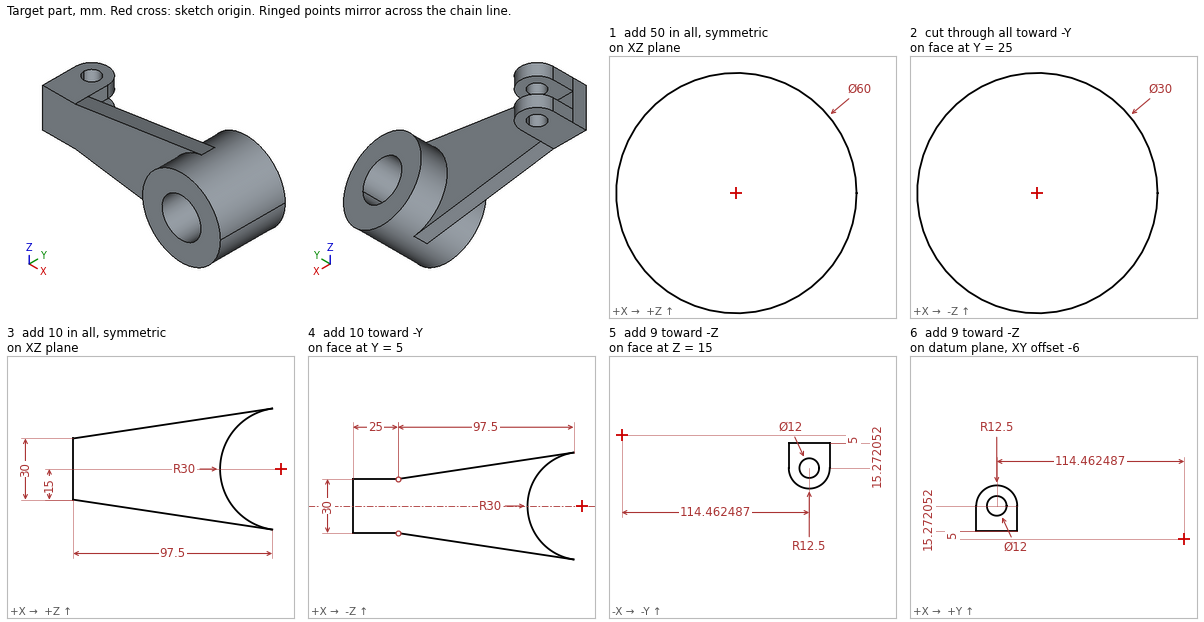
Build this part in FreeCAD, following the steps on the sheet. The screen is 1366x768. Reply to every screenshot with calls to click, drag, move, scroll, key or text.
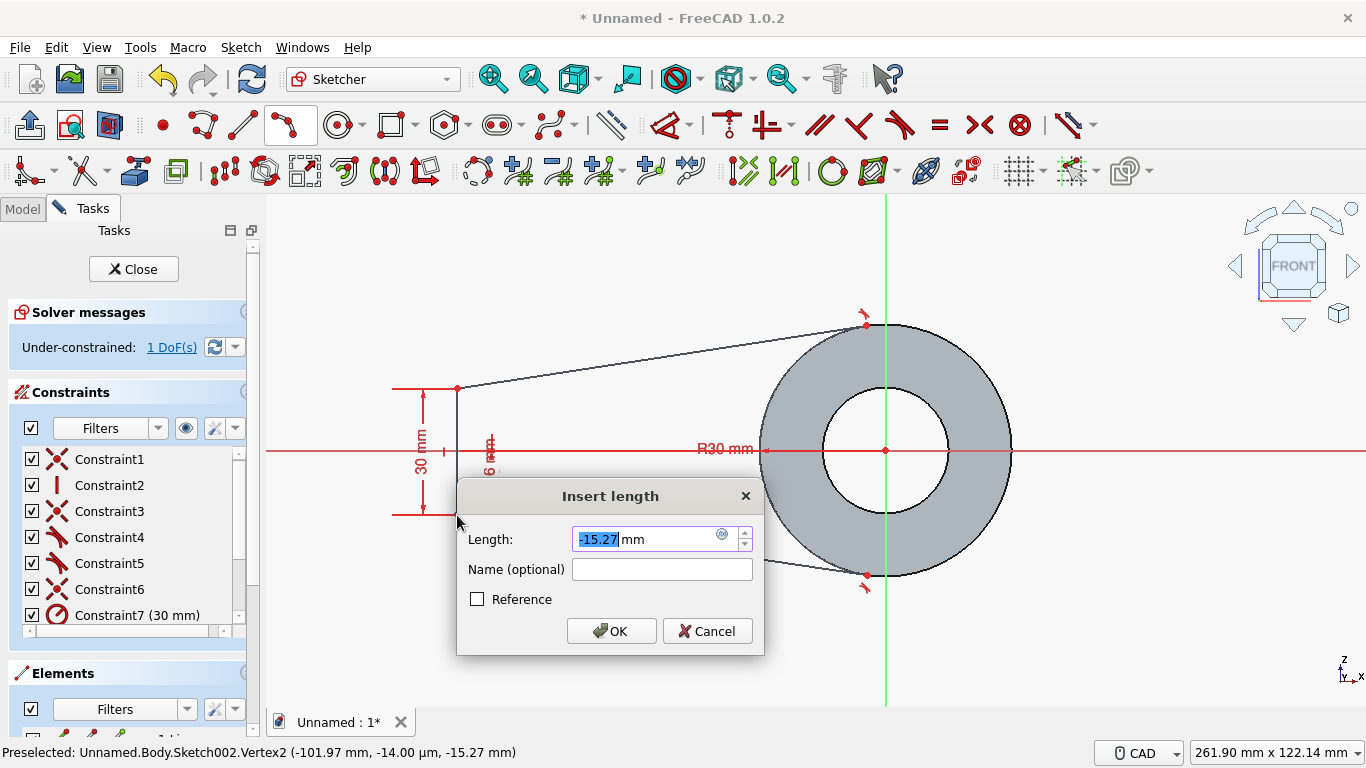
text(-15)
key(Return)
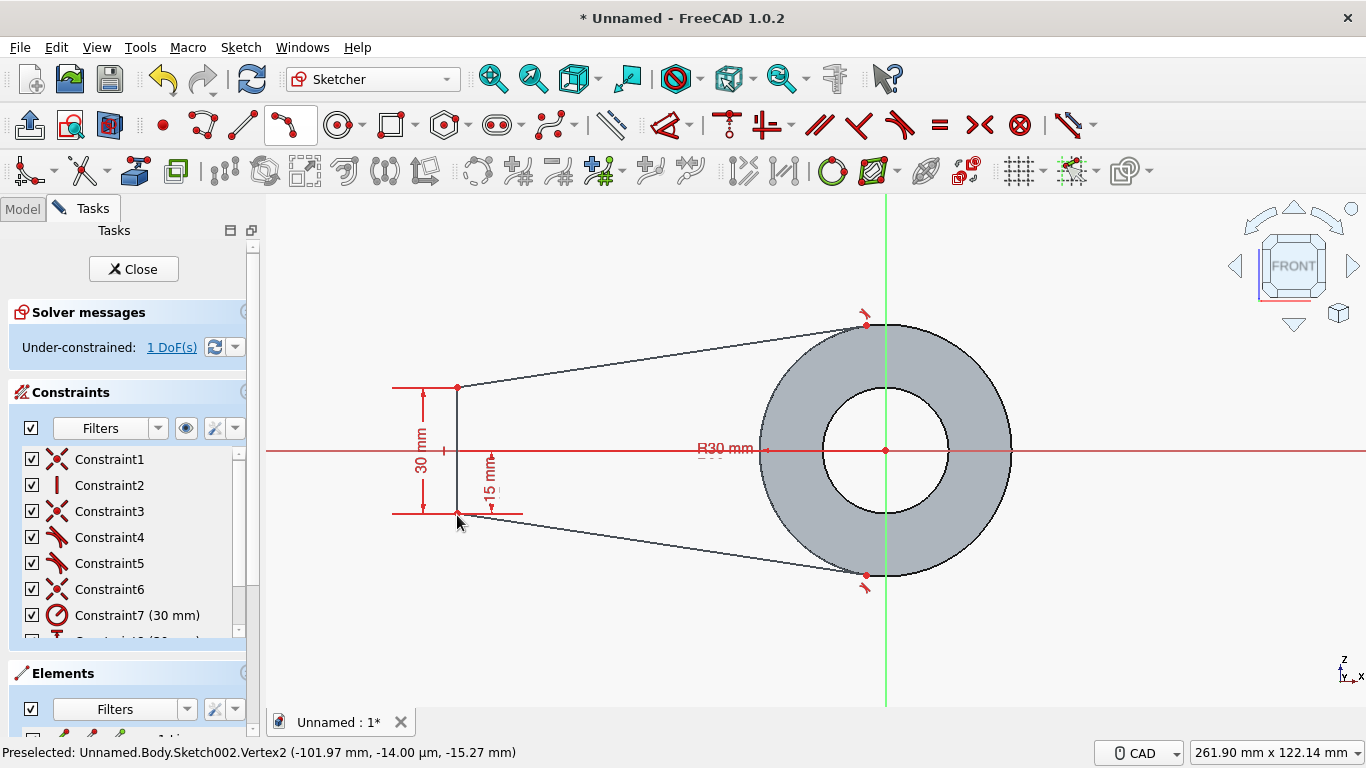
click(744, 557)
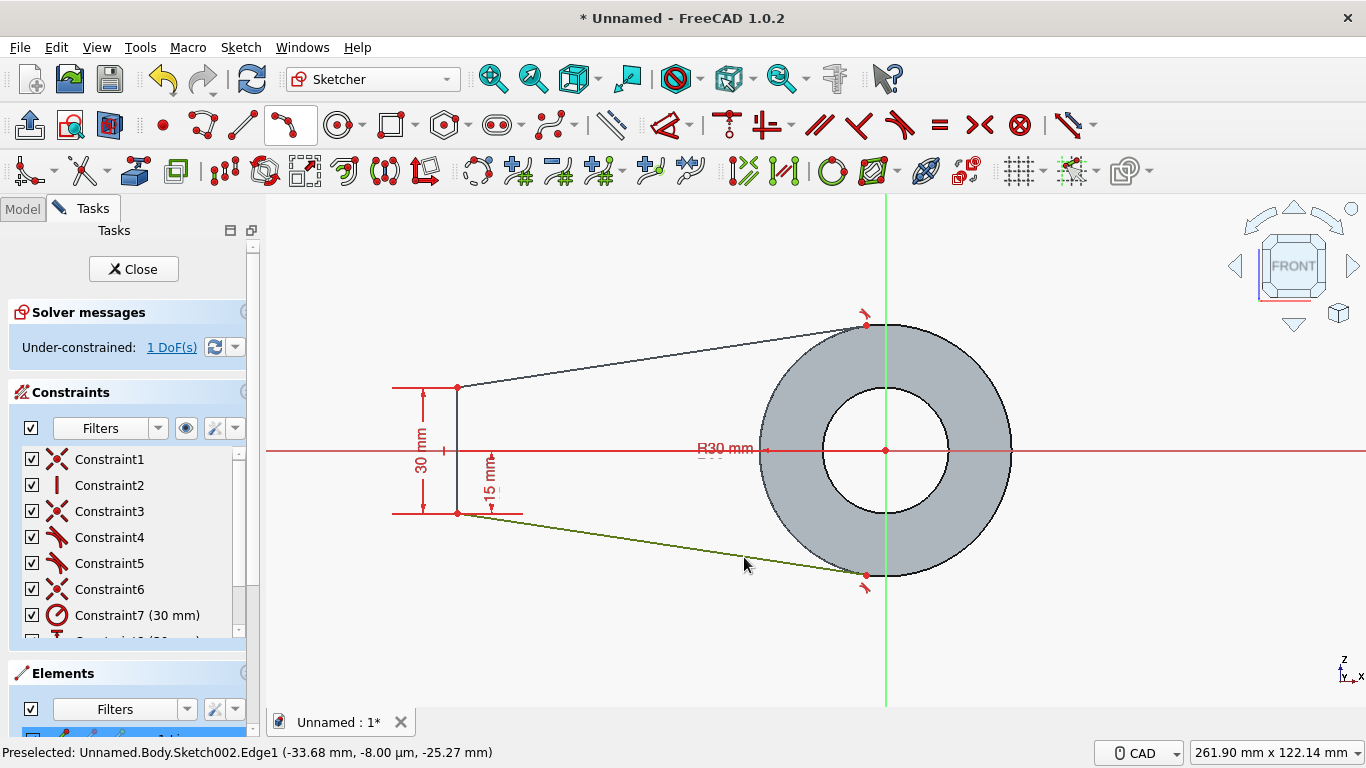
click(692, 126)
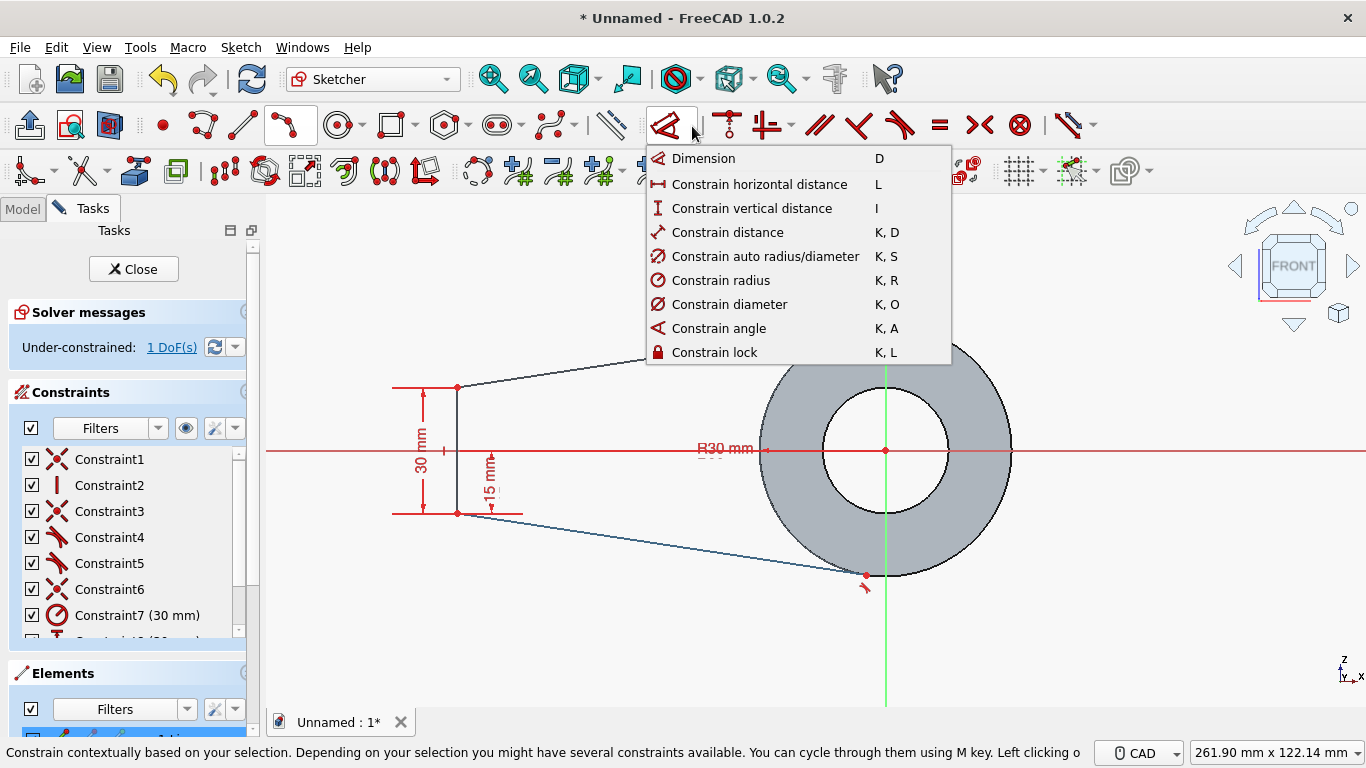
click(799, 184)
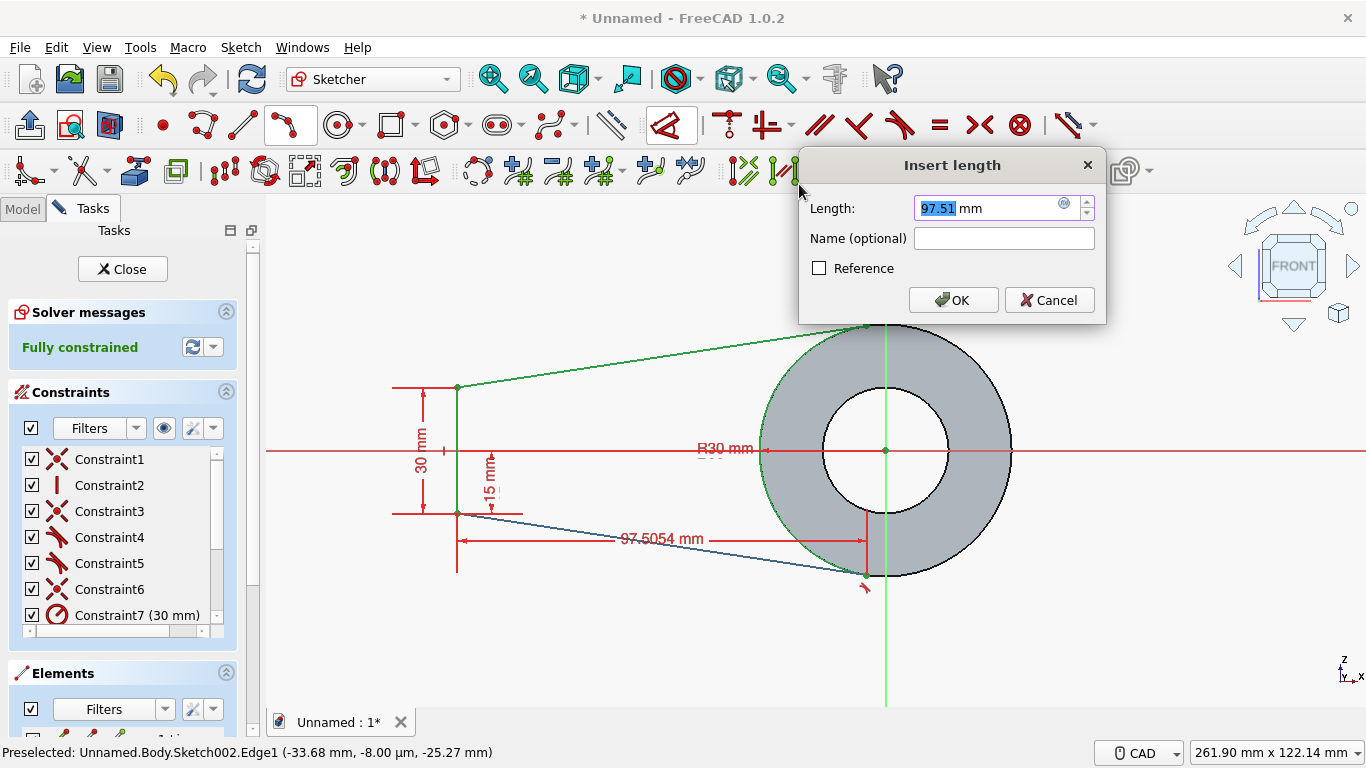
text(97.5)
key(Return)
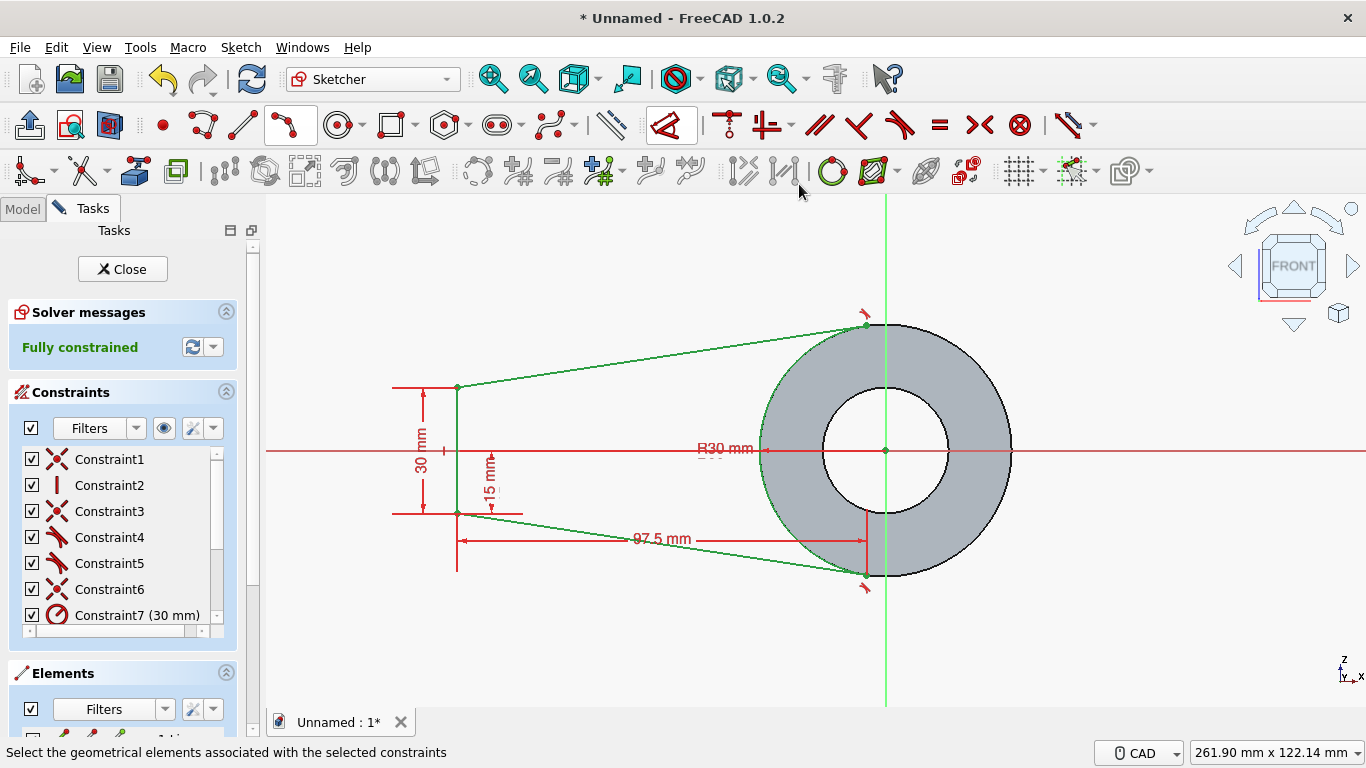
click(123, 269)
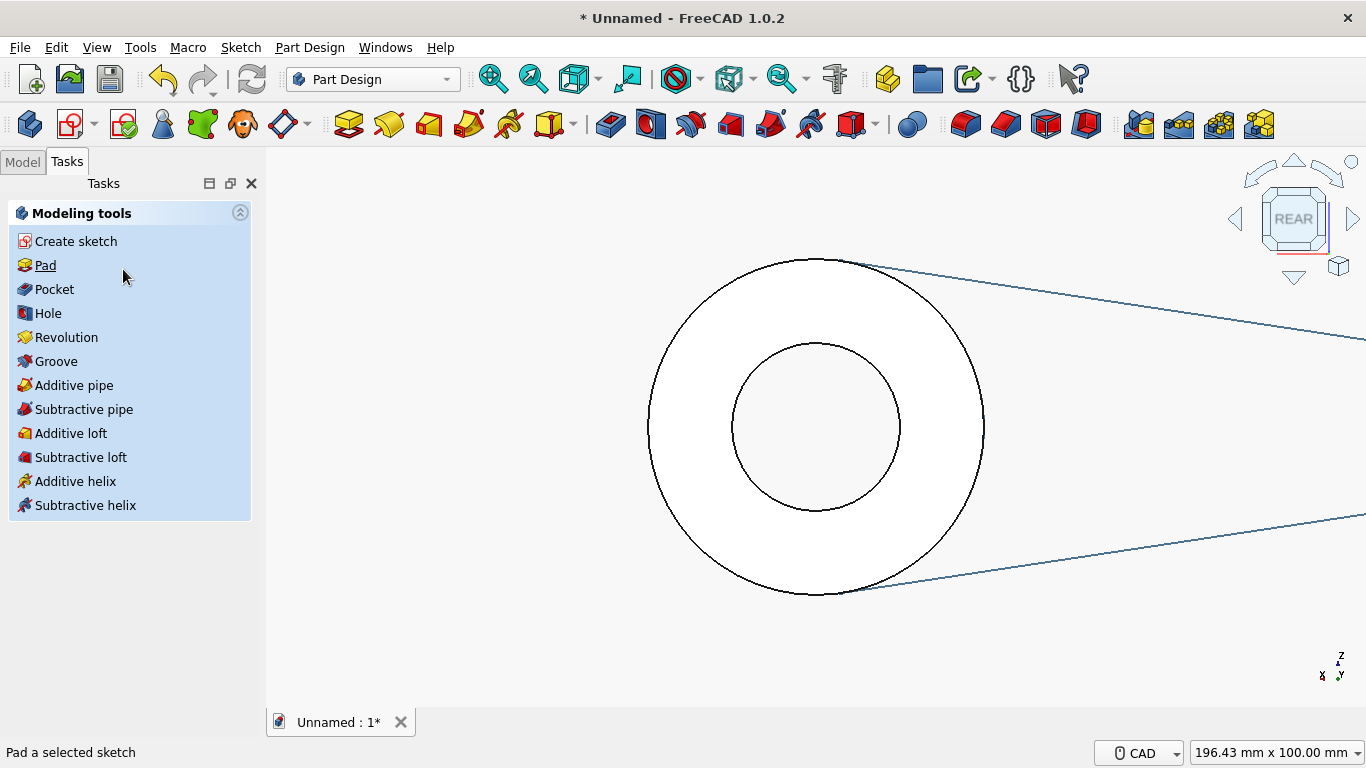
click(350, 124)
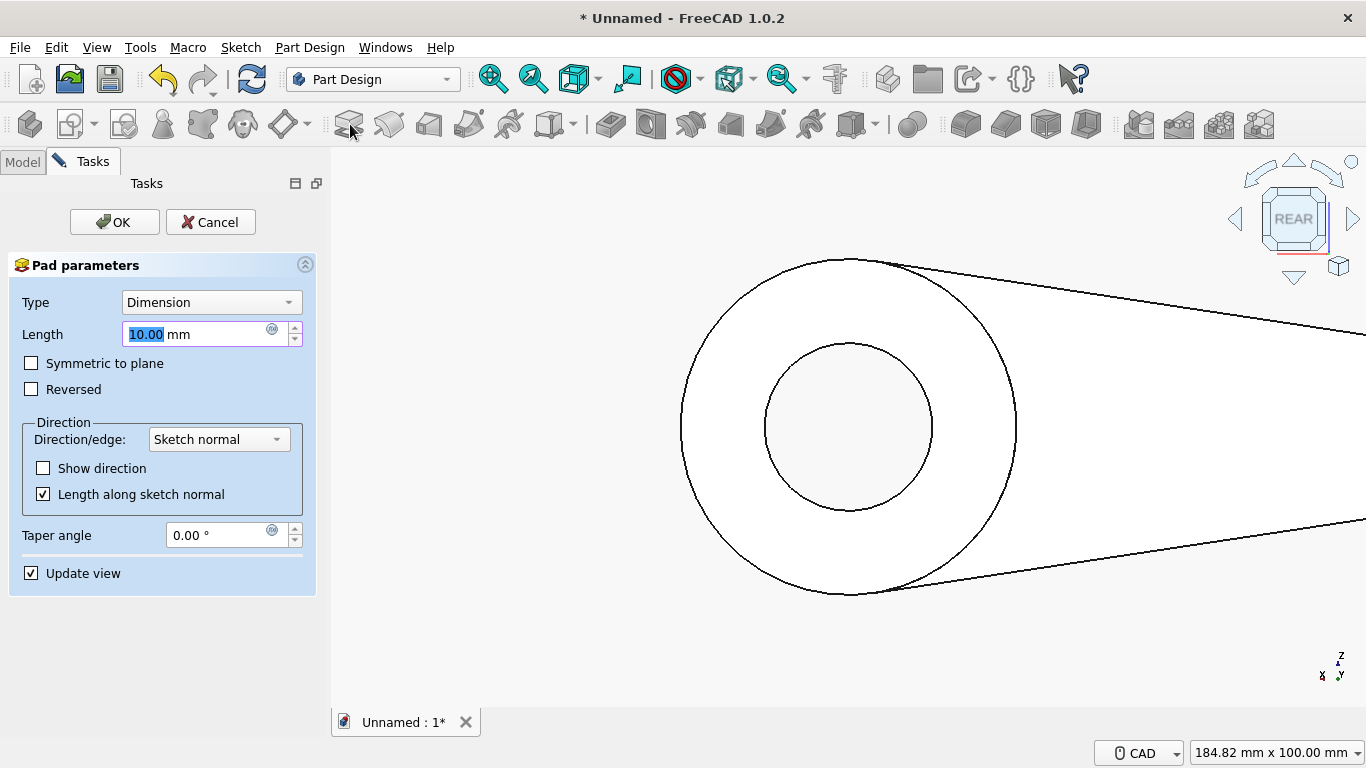
text(10)
key(Tab)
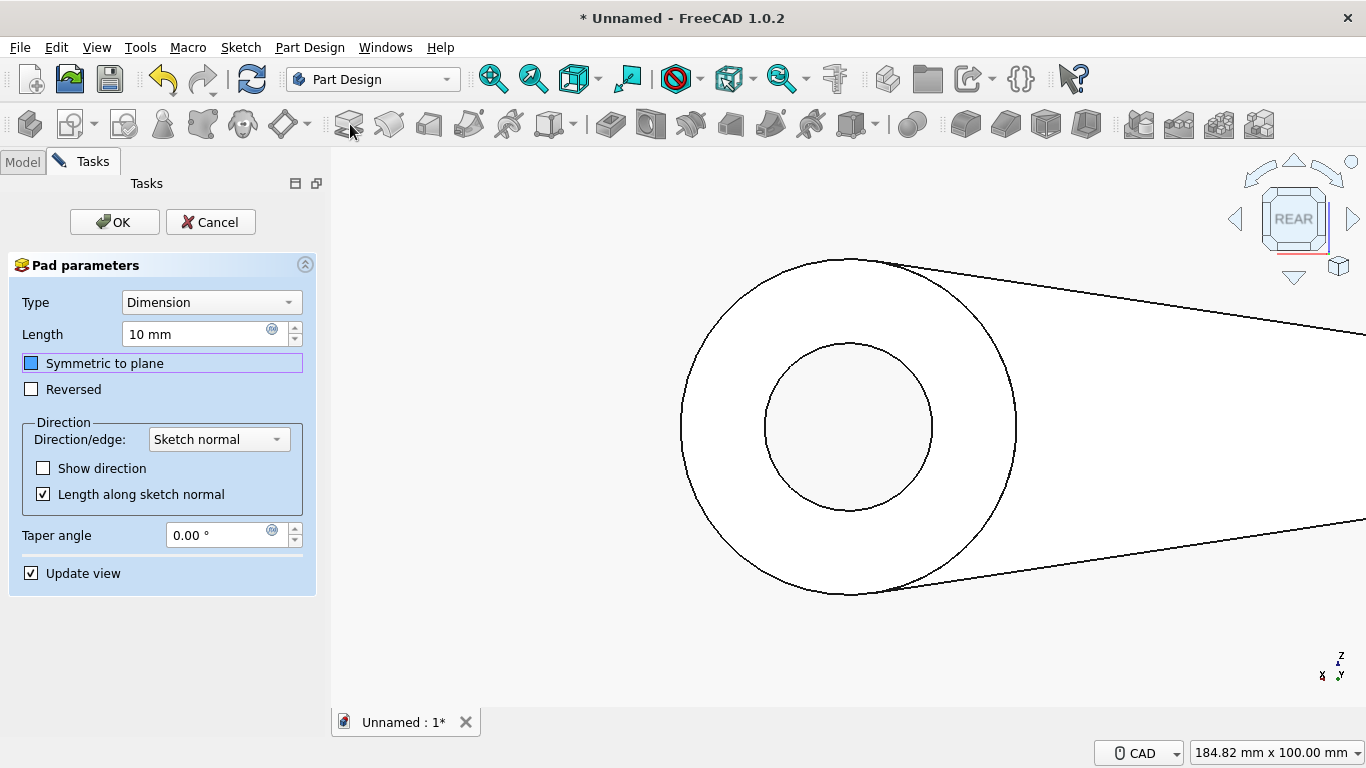
click(30, 363)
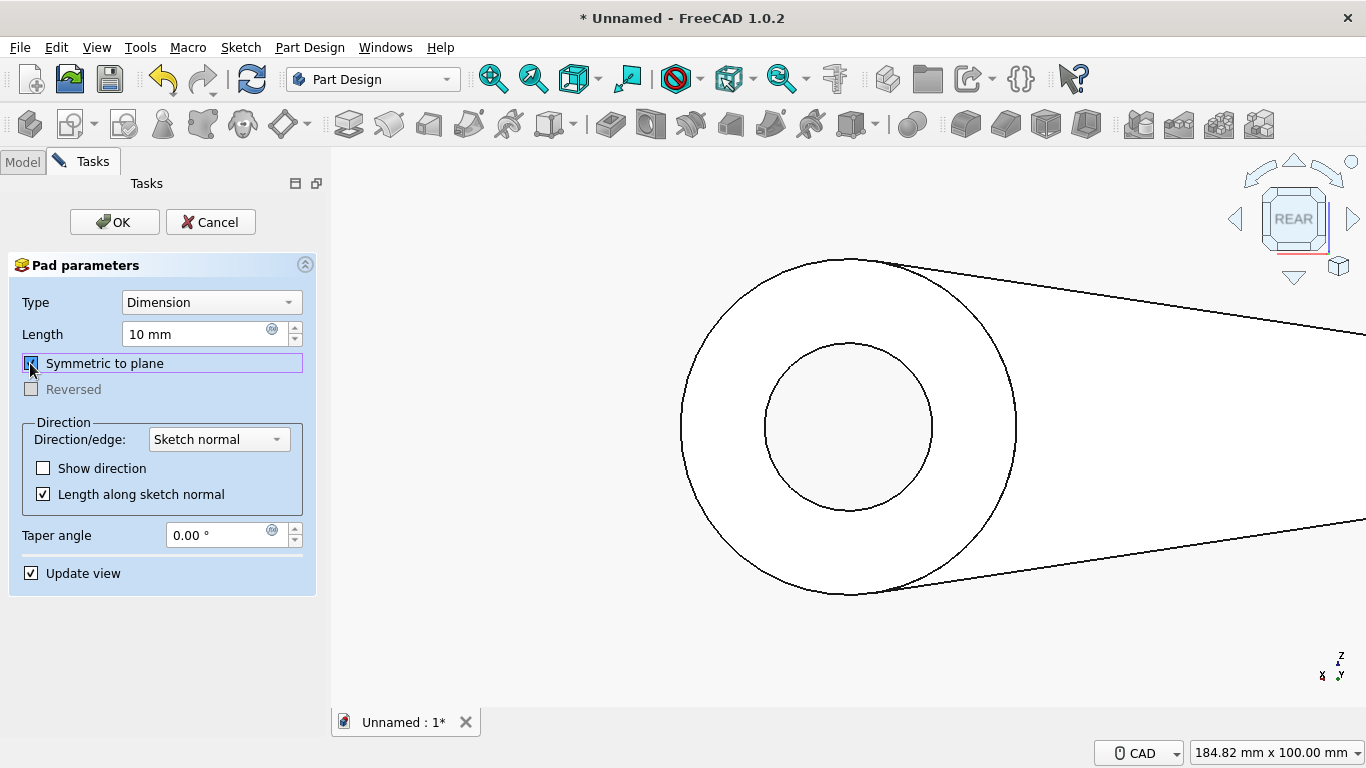
click(115, 222)